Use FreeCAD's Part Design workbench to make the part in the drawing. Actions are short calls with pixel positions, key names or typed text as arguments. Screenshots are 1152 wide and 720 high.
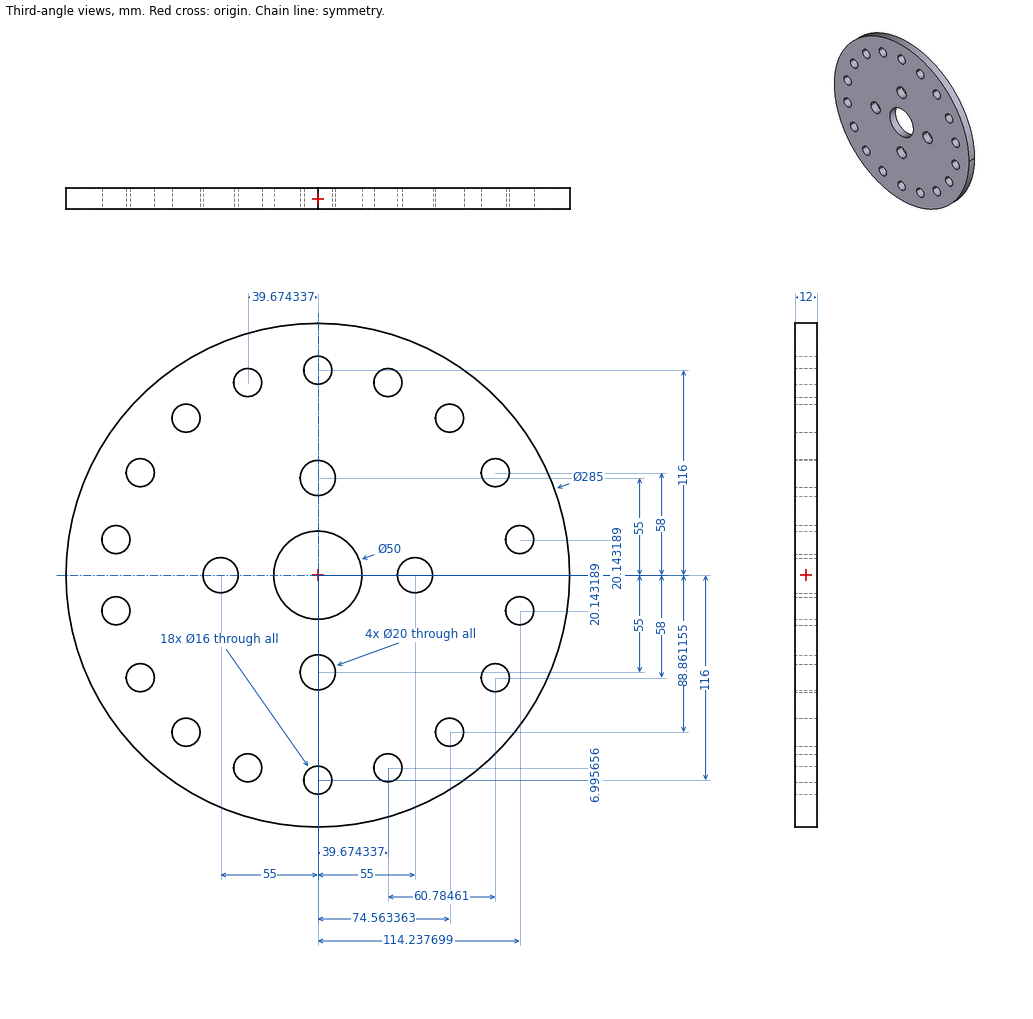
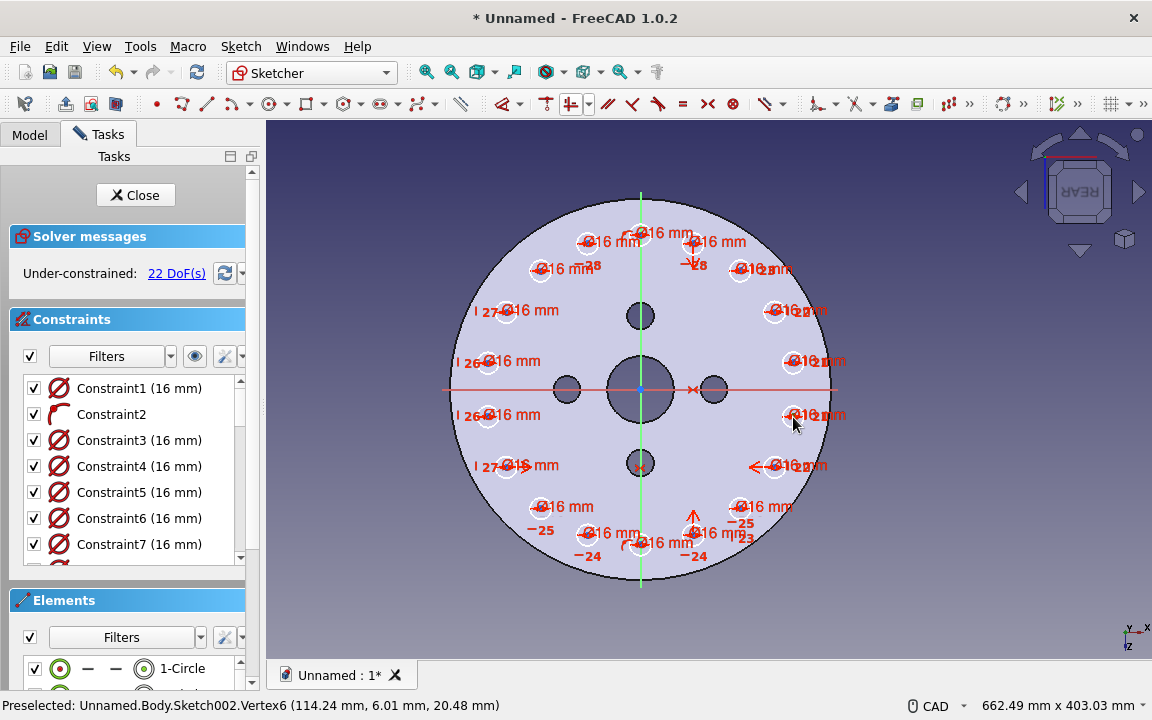
click(488, 417)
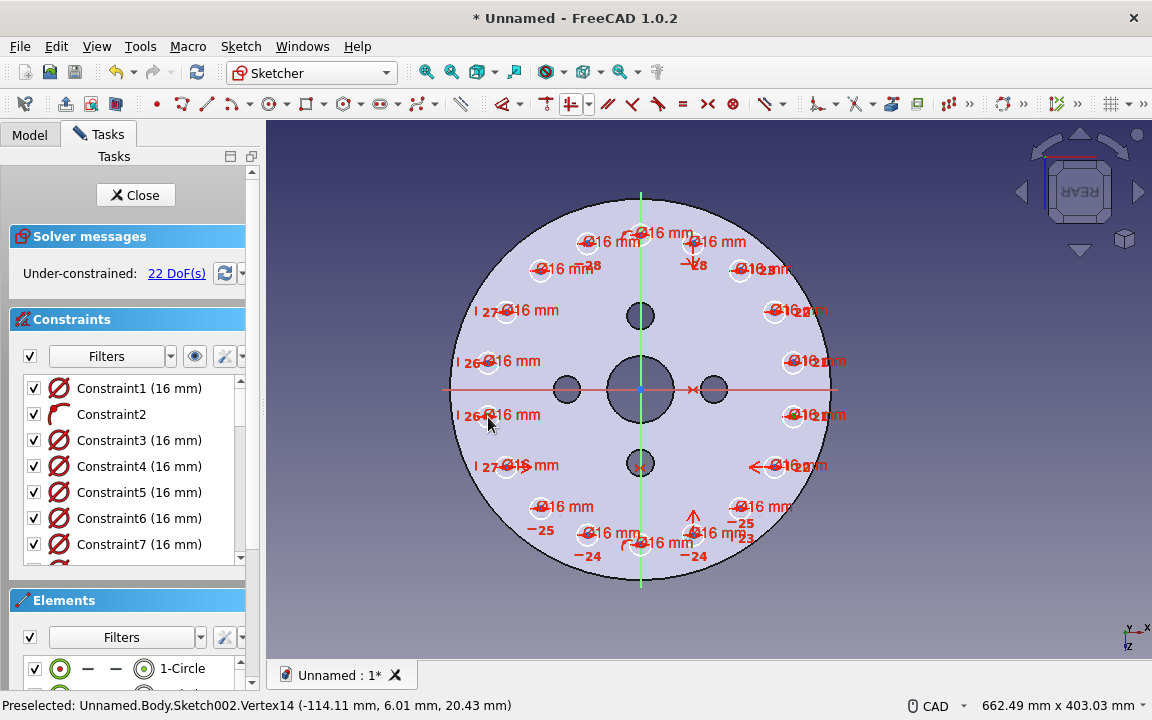
click(641, 493)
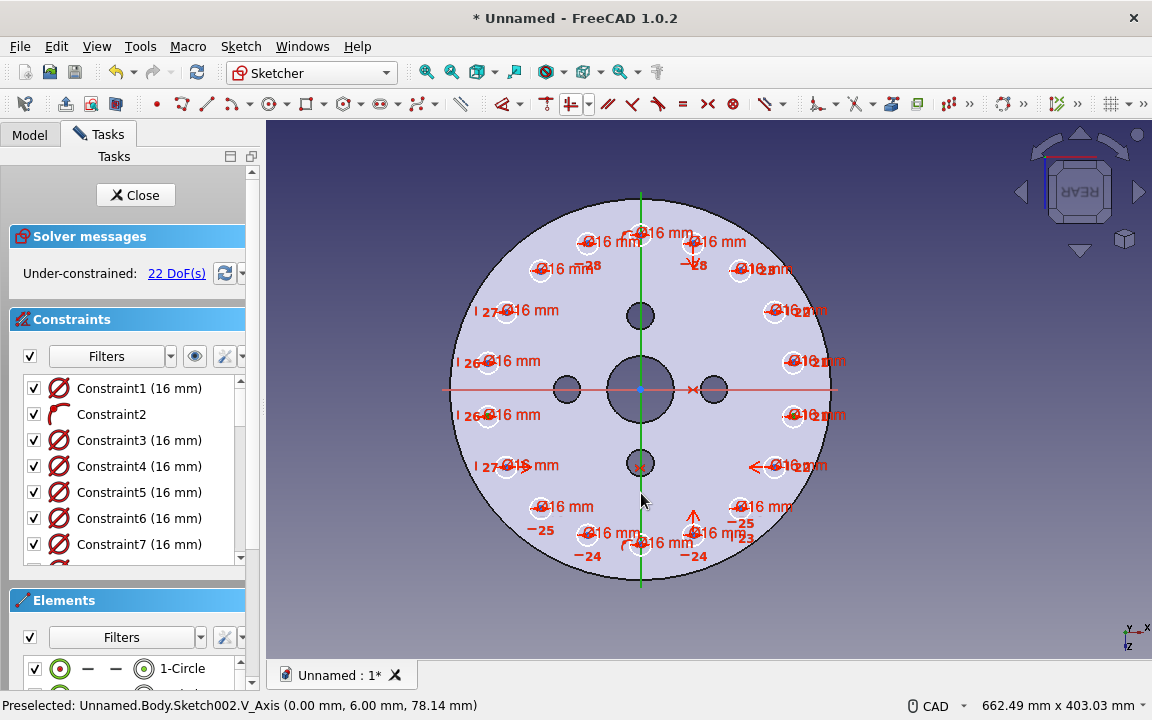
key(s)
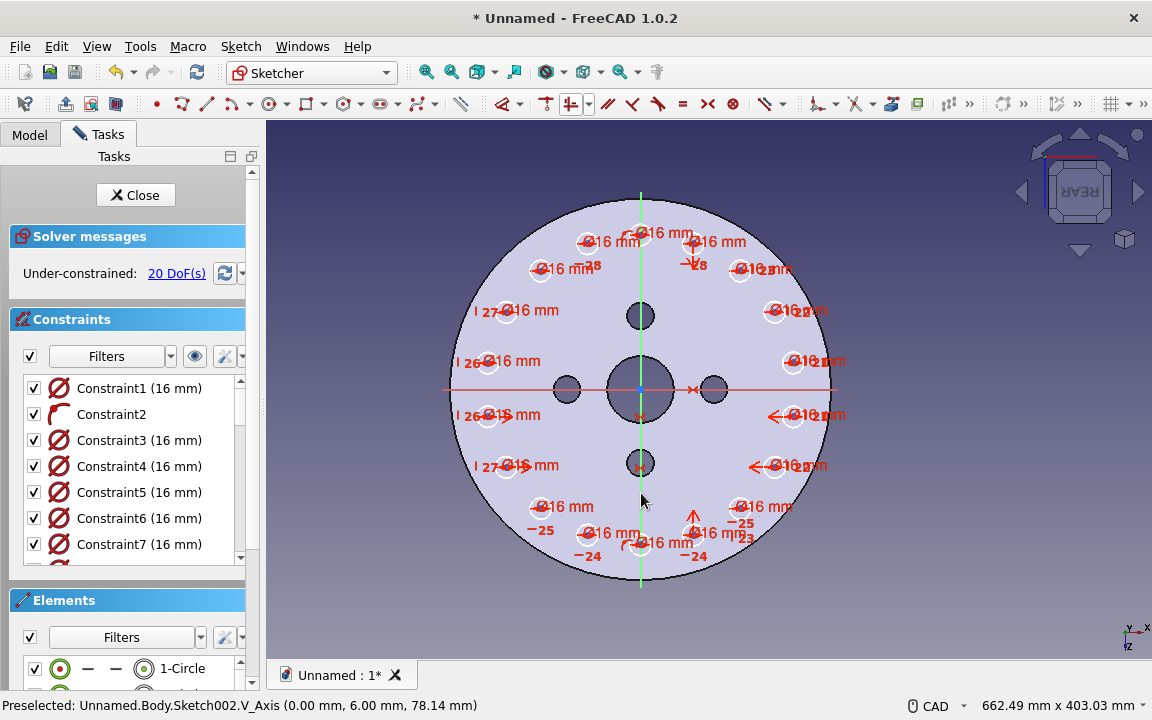
click(740, 271)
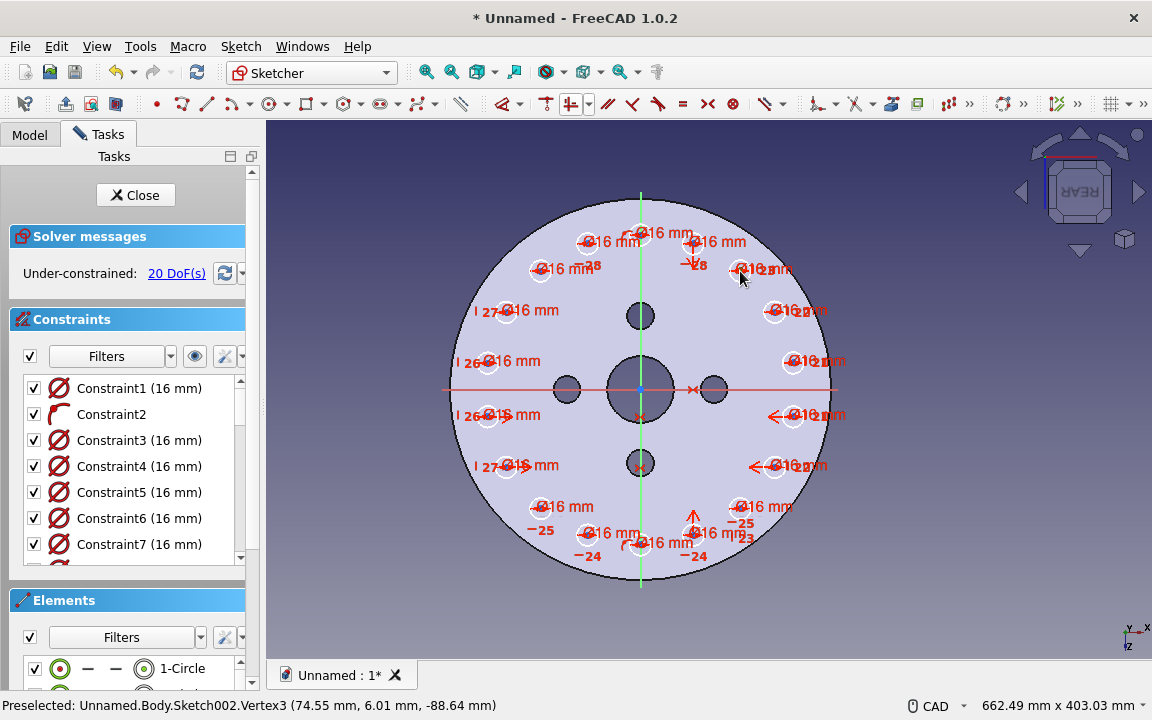
click(541, 271)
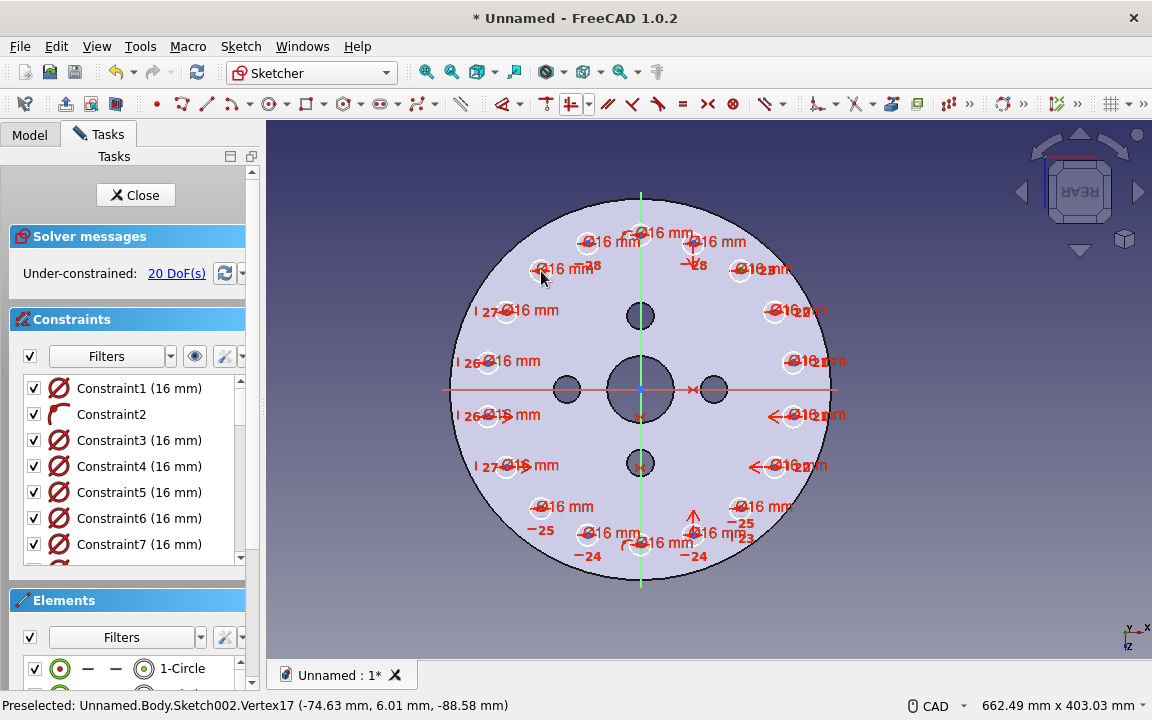
click(641, 493)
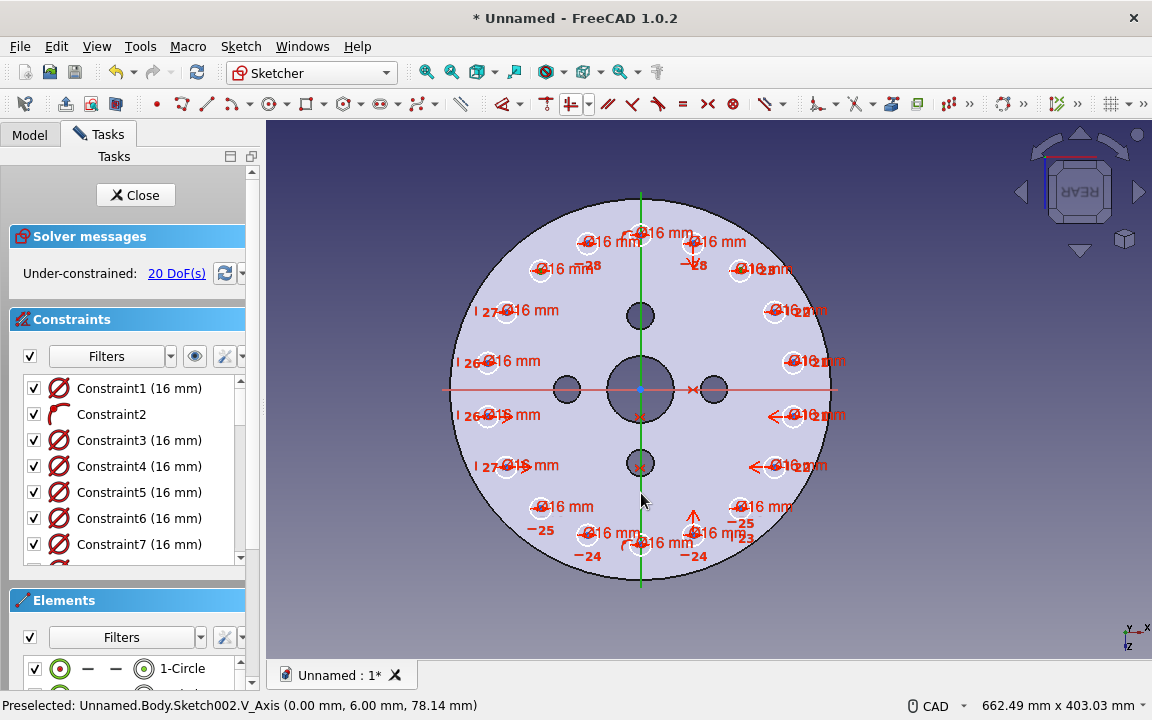
key(s)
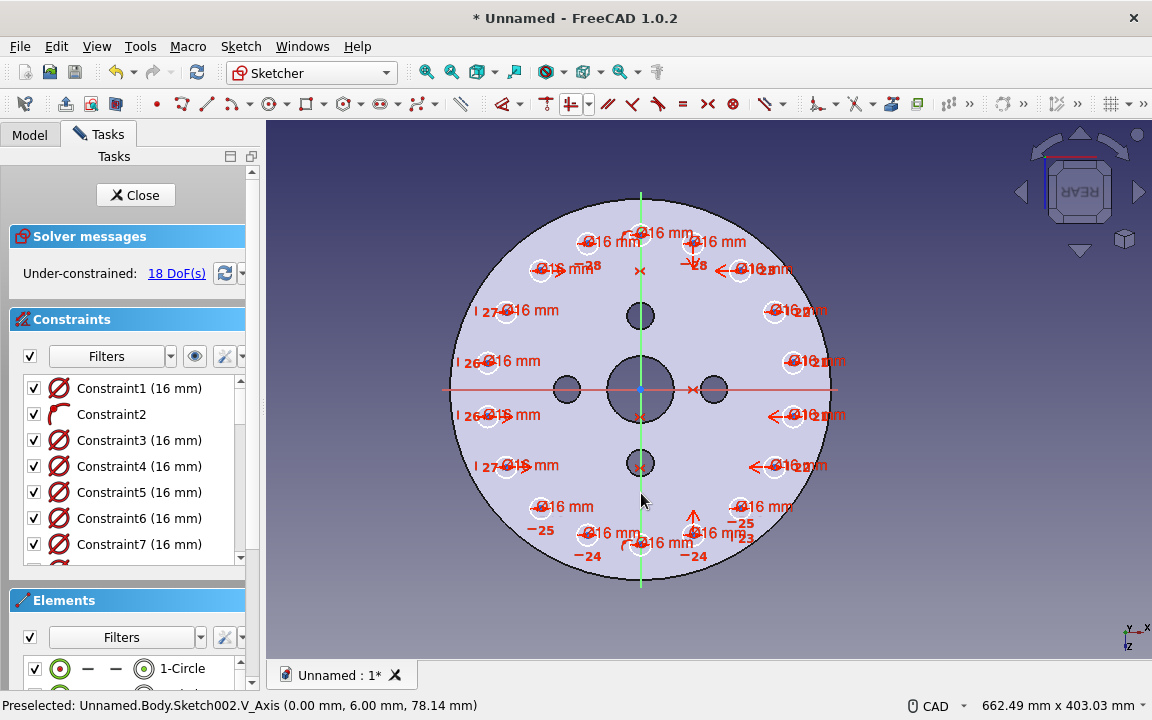
click(541, 509)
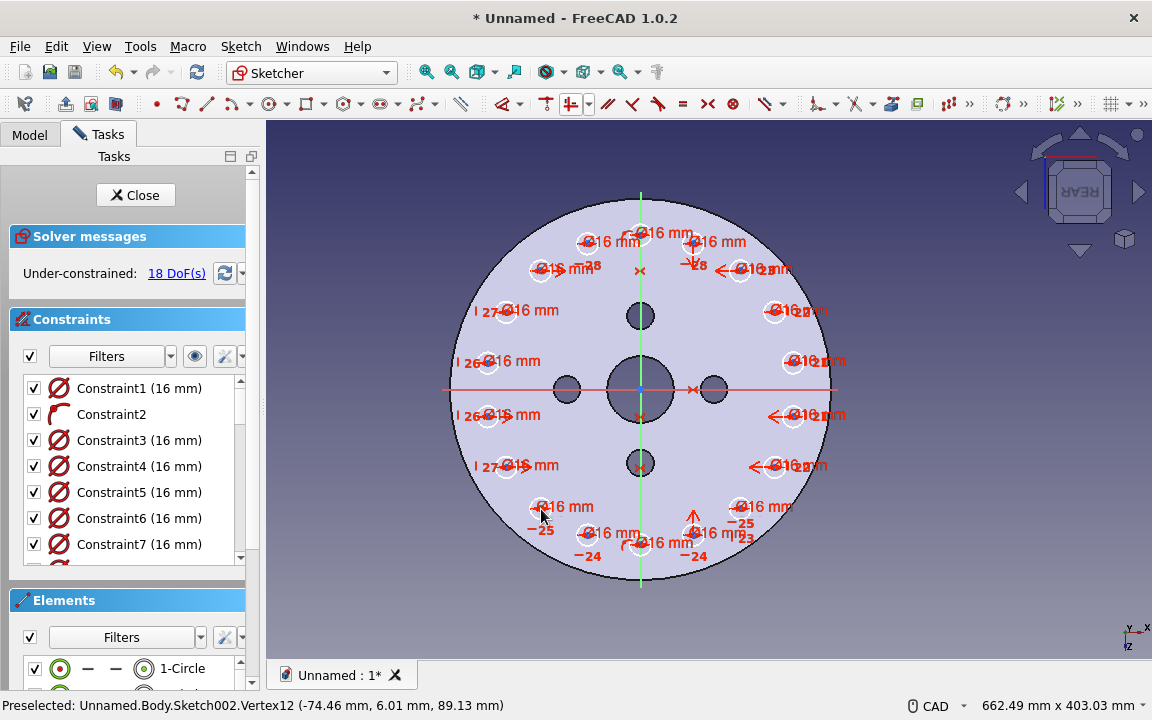
click(541, 271)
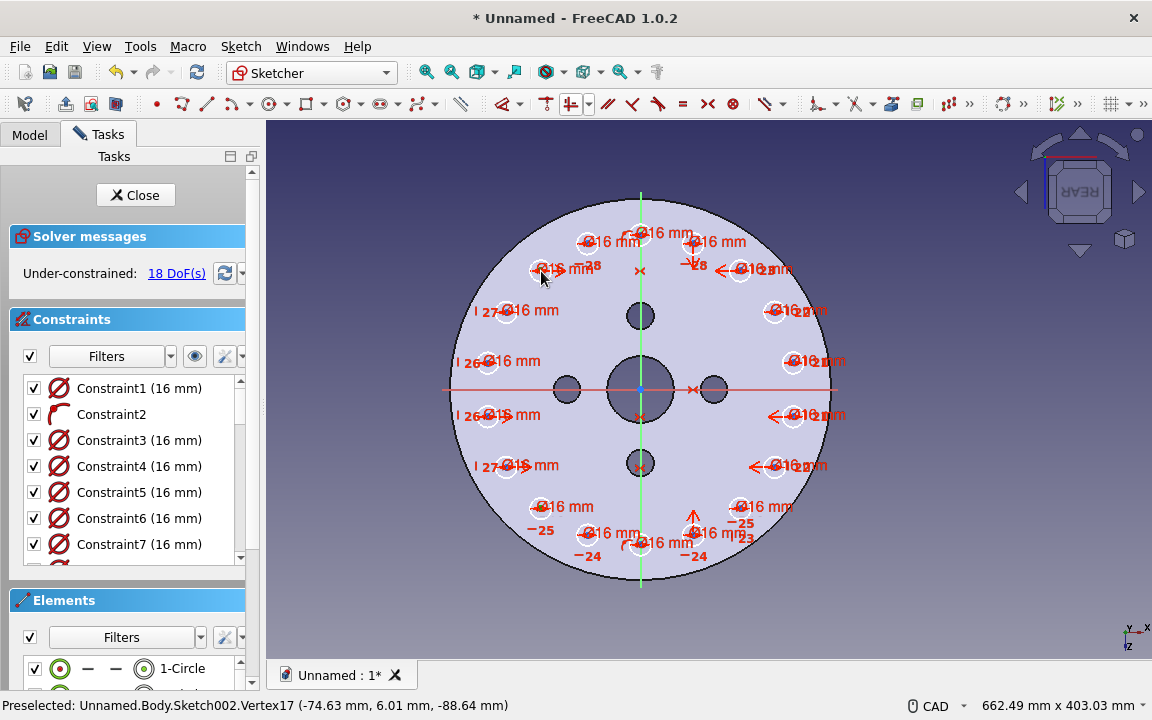
click(442, 389)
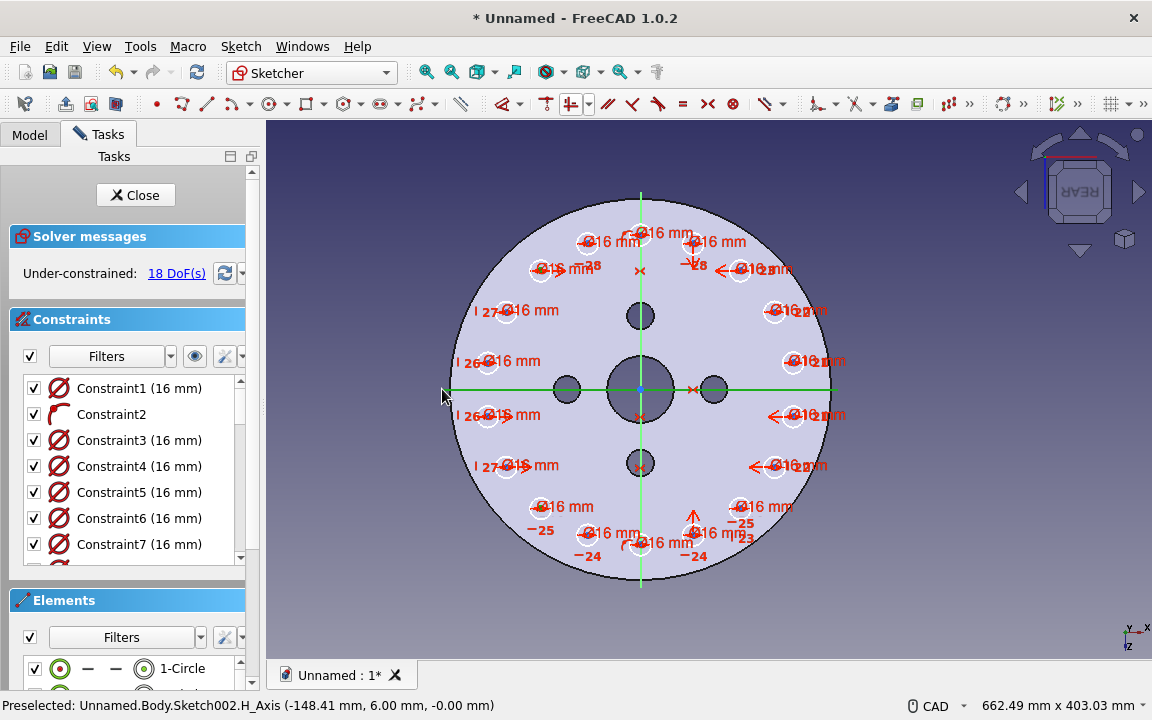
key(s)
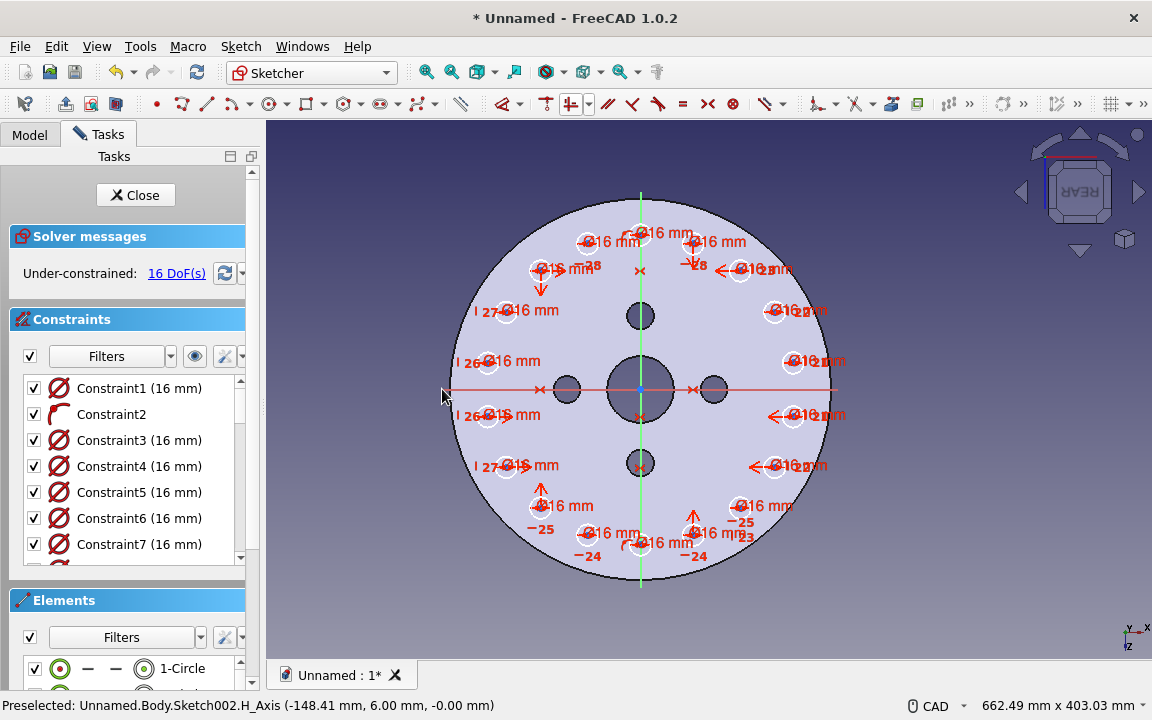
click(502, 104)